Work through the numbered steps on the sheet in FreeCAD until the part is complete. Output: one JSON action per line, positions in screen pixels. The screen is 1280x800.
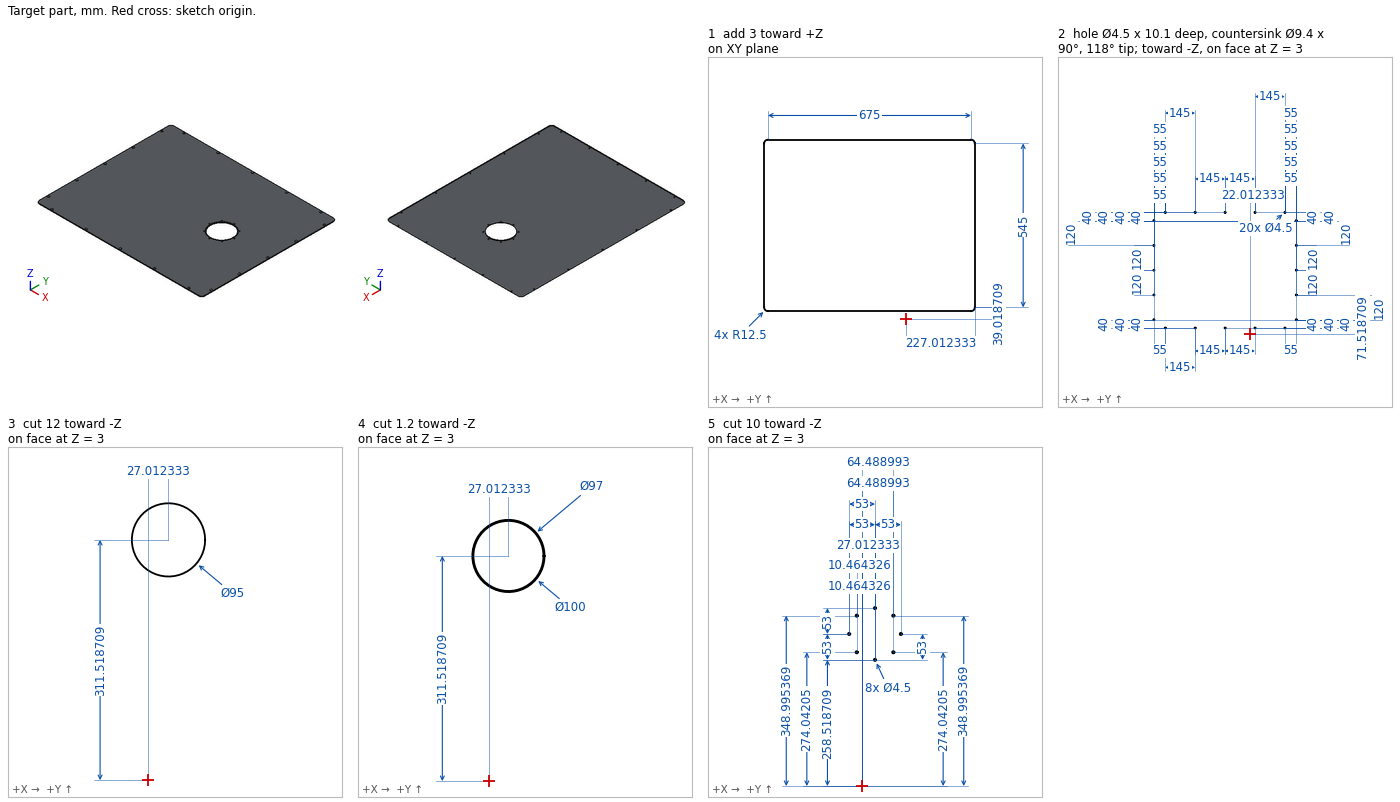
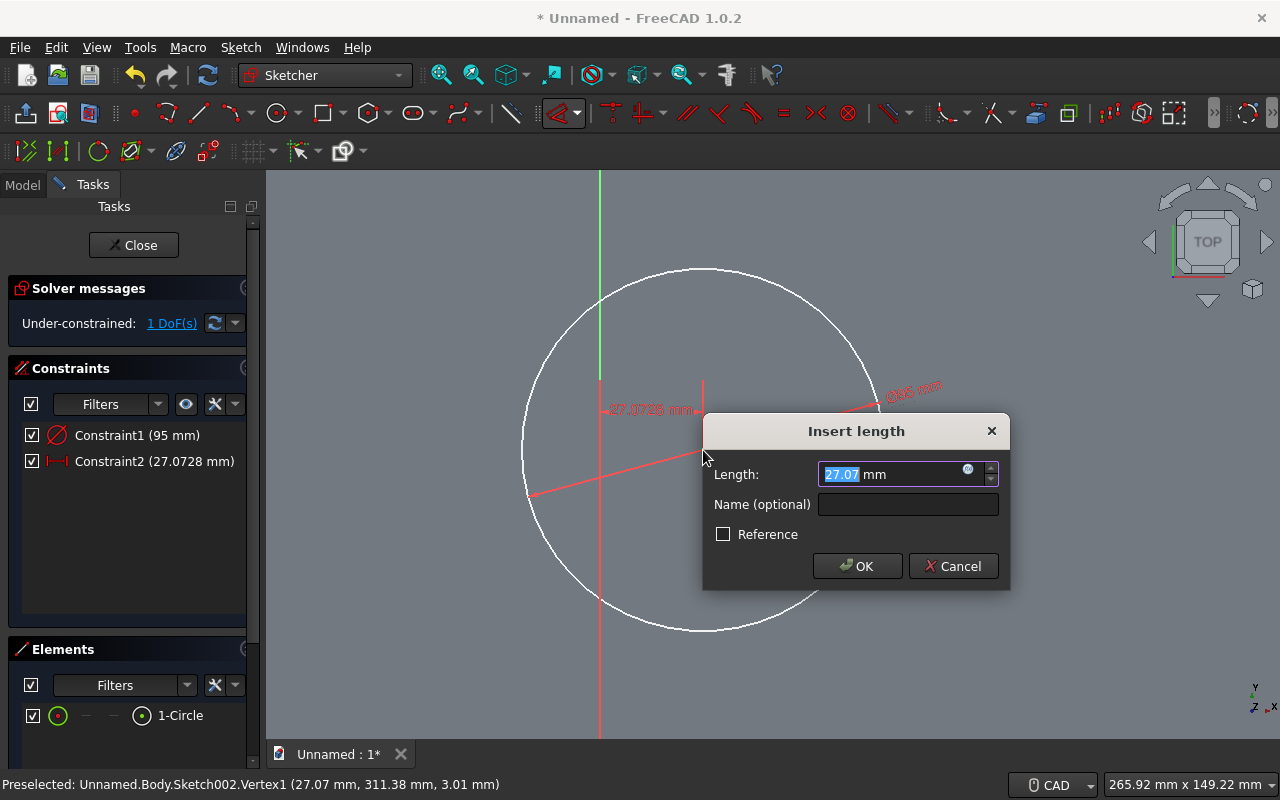
{"action": "type", "text": "27.012333"}
{"action": "key", "text": "Return"}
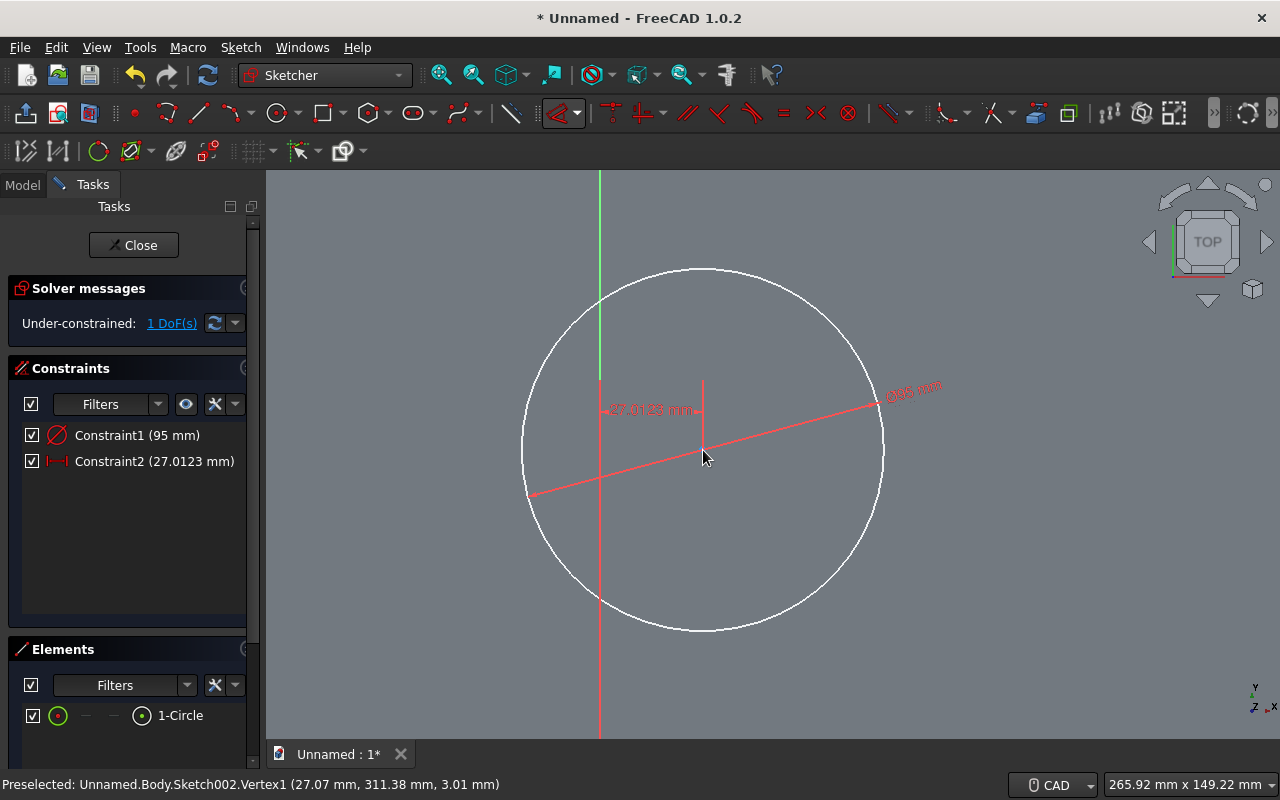
{"action": "left_click", "coordinate": [703, 450]}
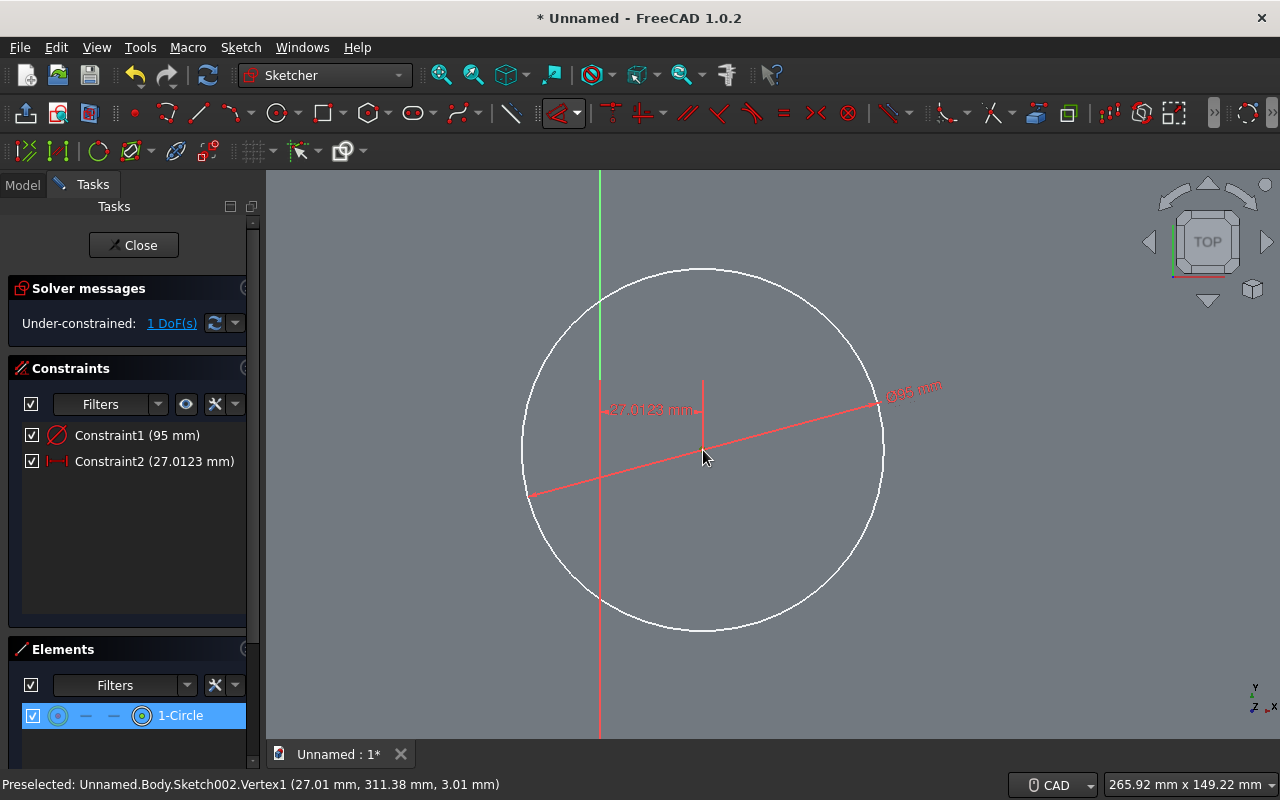
{"action": "left_click", "coordinate": [580, 114]}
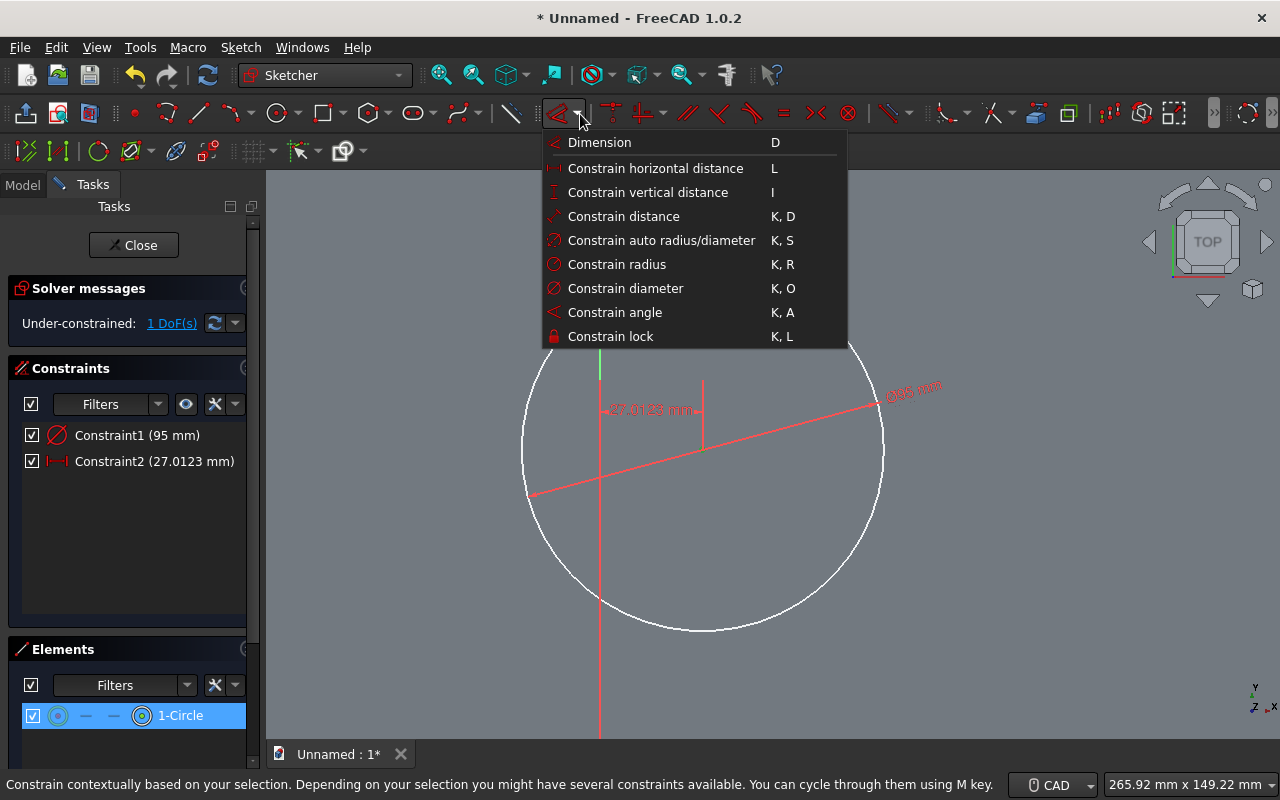
{"action": "left_click", "coordinate": [695, 192]}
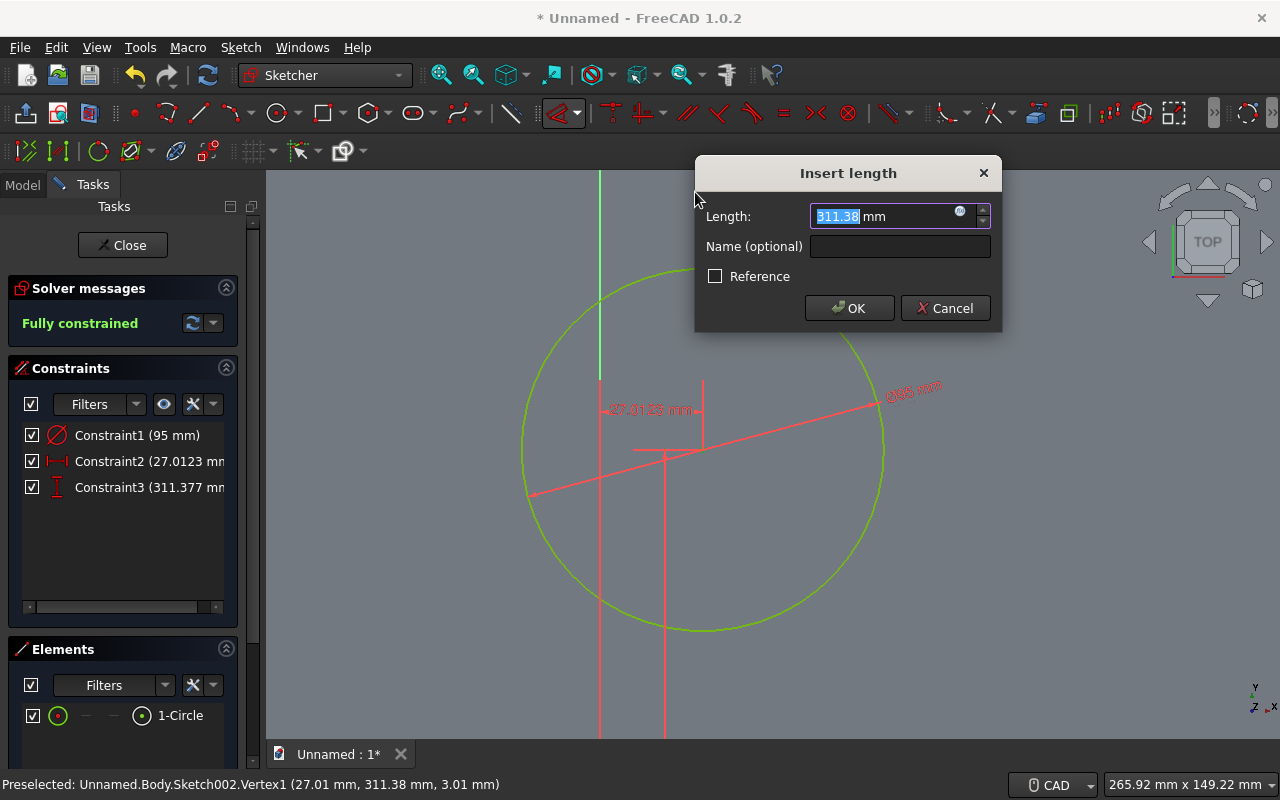
{"action": "type", "text": "311.518709"}
{"action": "key", "text": "Return"}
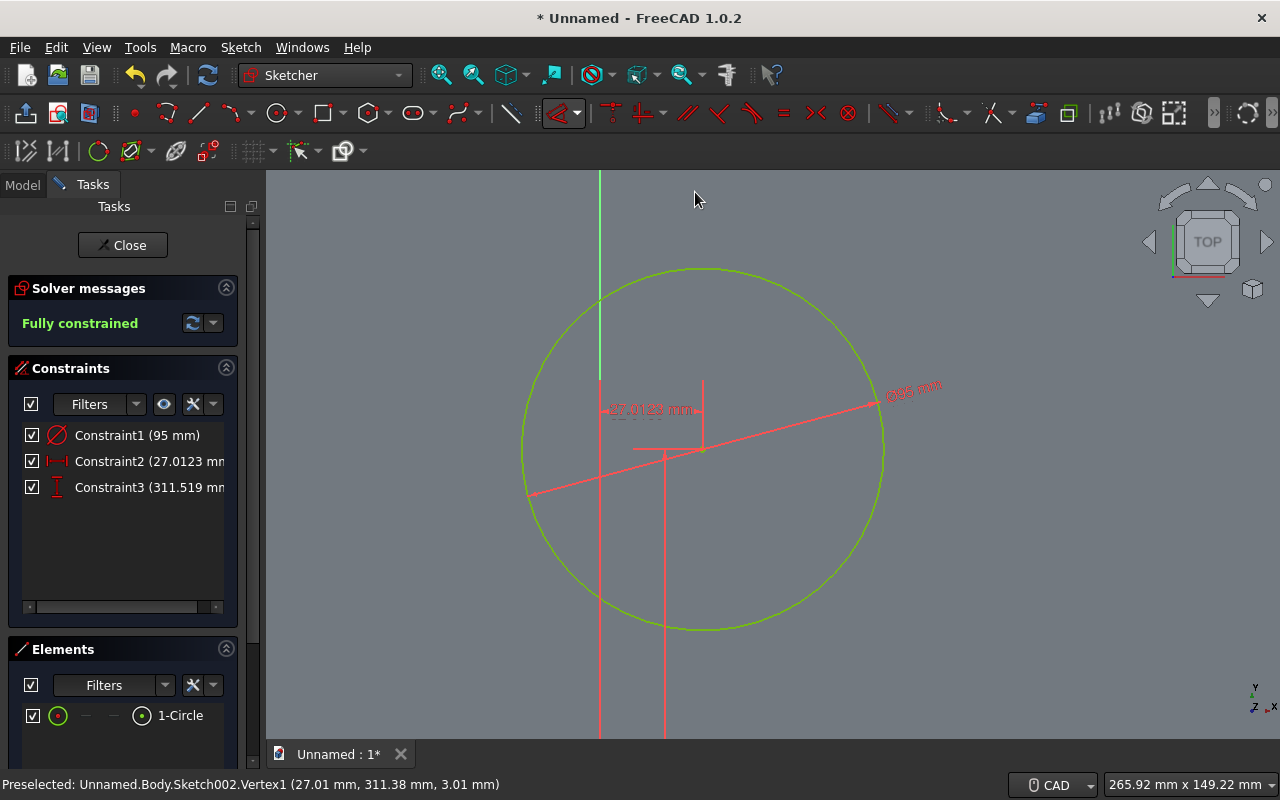
{"action": "left_click", "coordinate": [123, 245]}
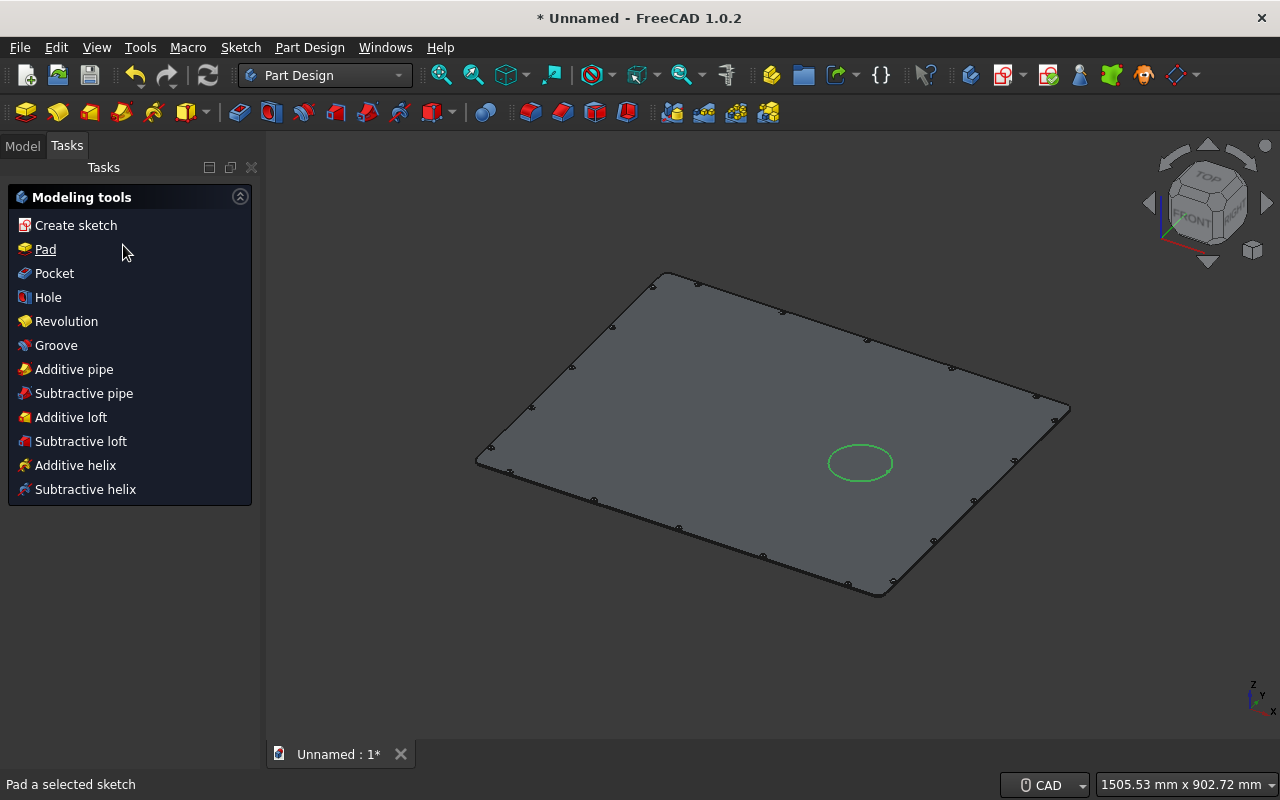
{"action": "left_click", "coordinate": [240, 112]}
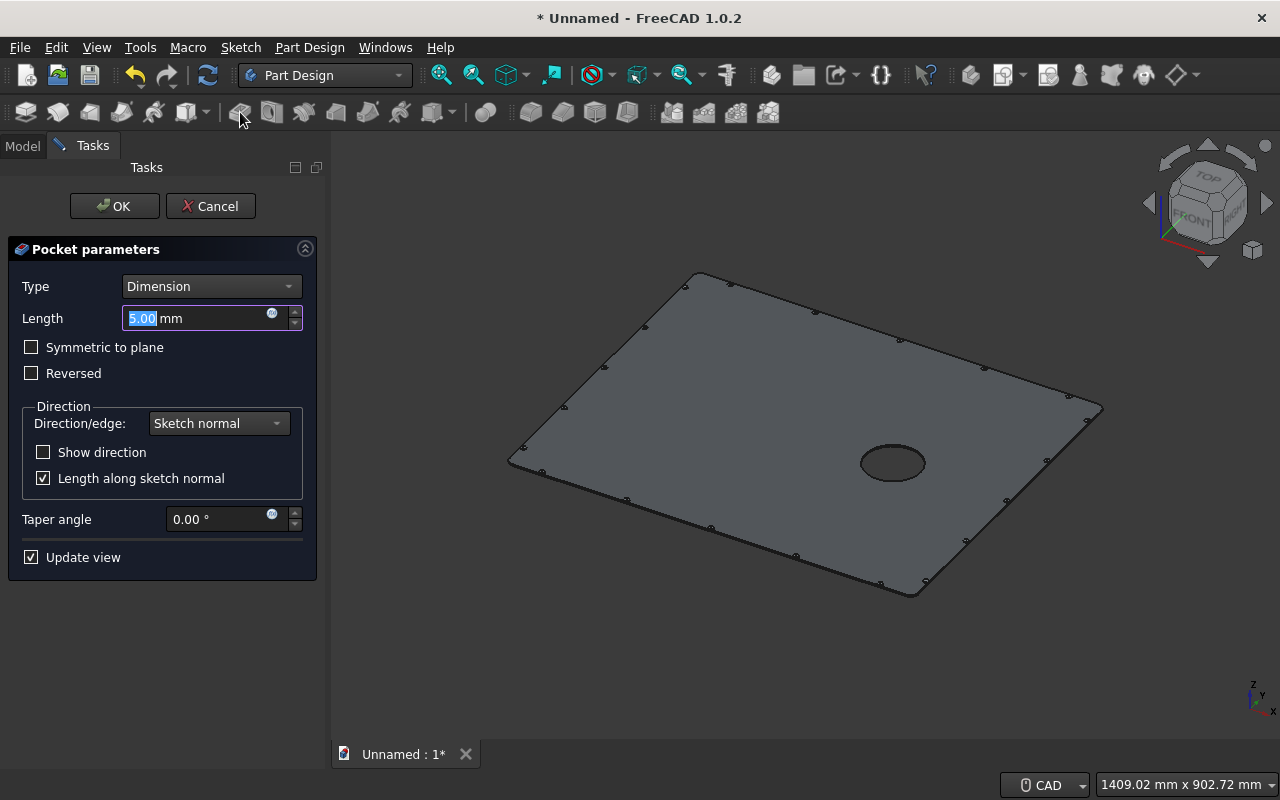
{"action": "type", "text": "12"}
{"action": "key", "text": "Tab"}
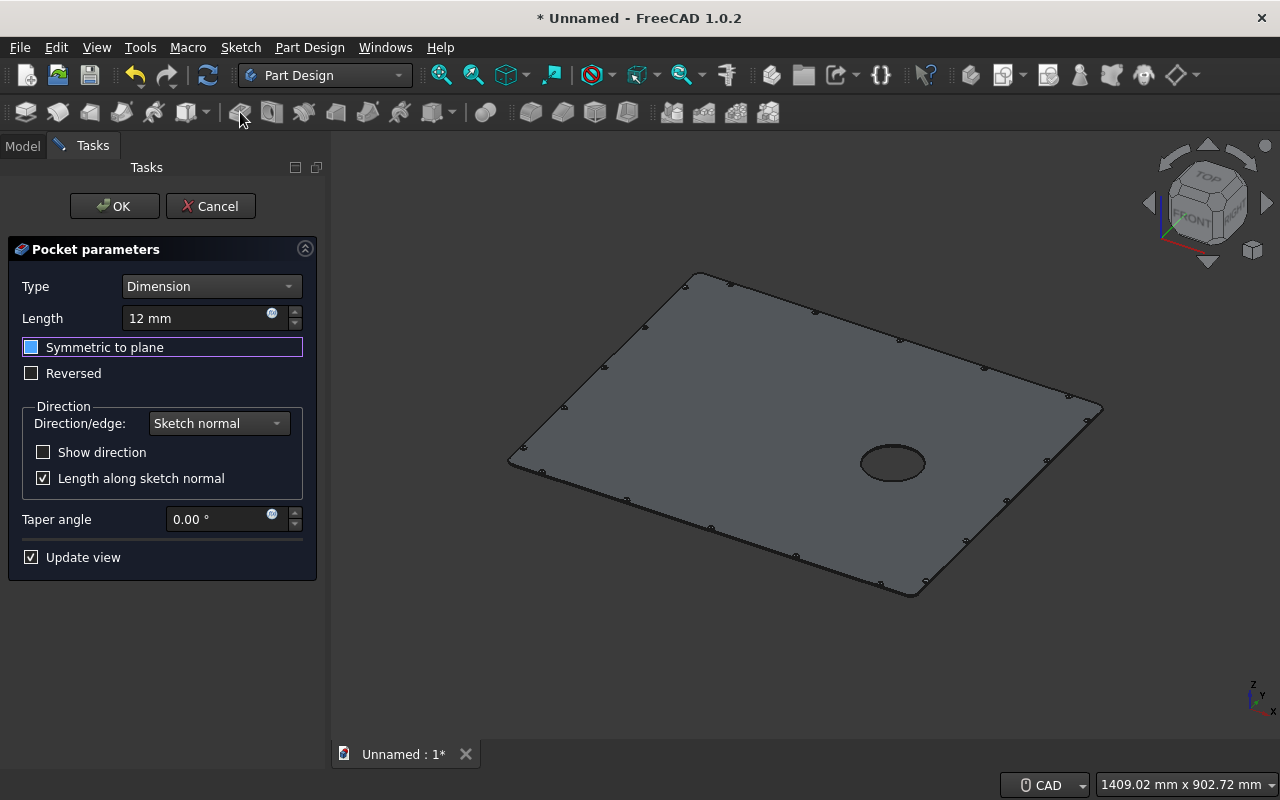
{"action": "left_click", "coordinate": [115, 206]}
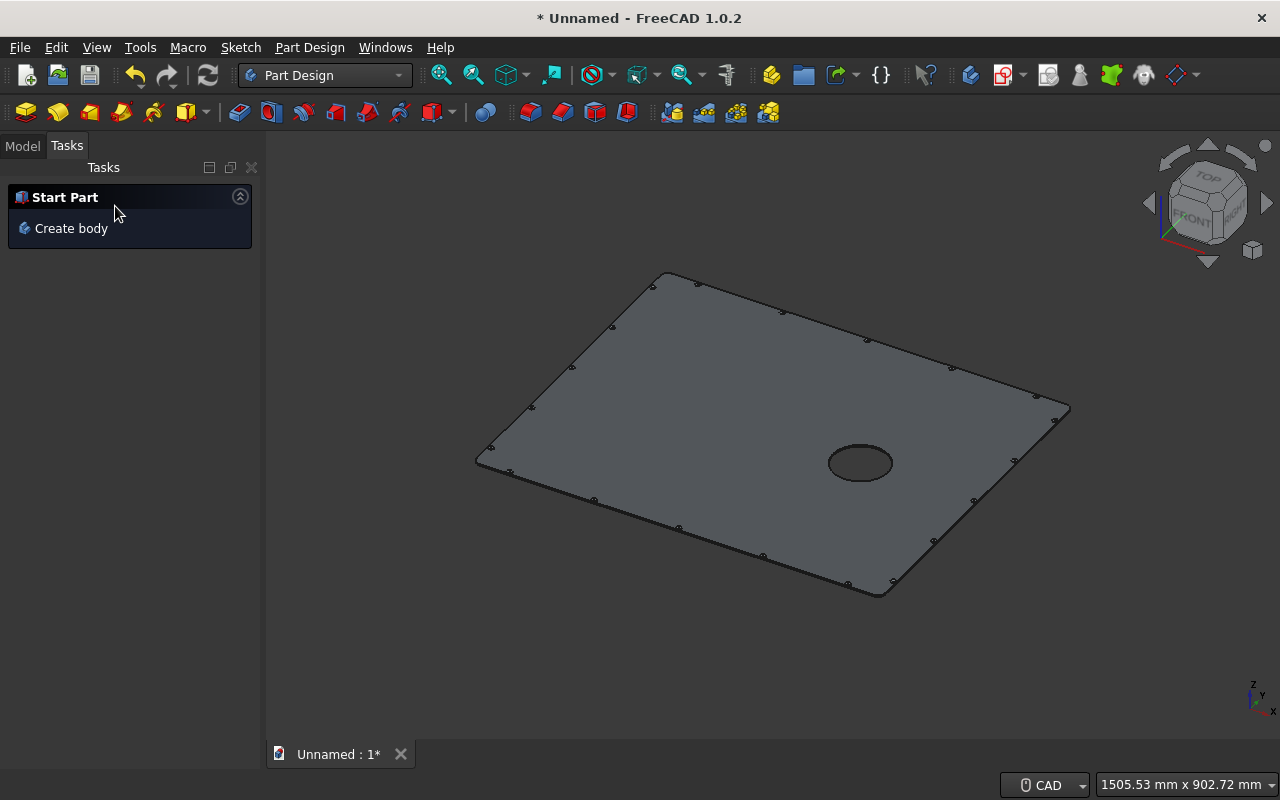
{"action": "left_click", "coordinate": [715, 414]}